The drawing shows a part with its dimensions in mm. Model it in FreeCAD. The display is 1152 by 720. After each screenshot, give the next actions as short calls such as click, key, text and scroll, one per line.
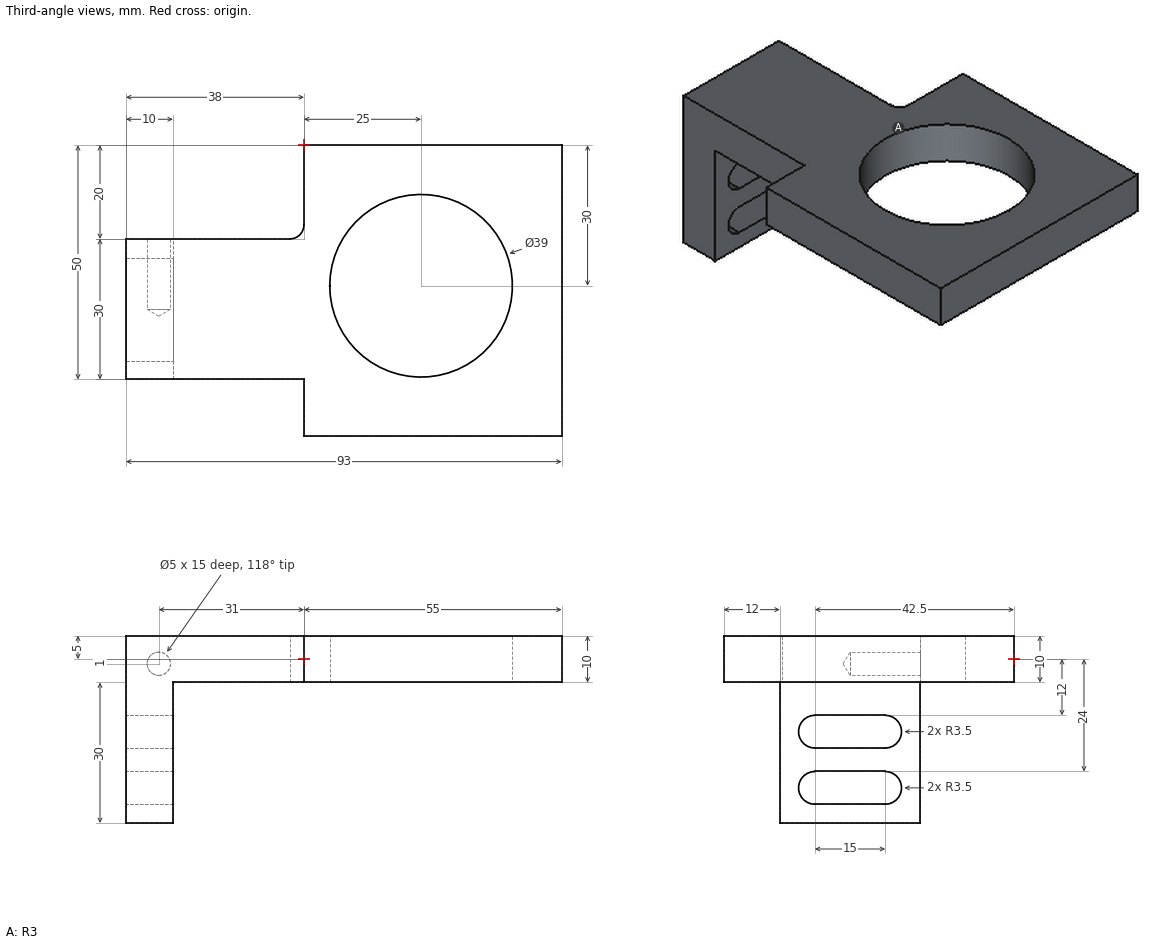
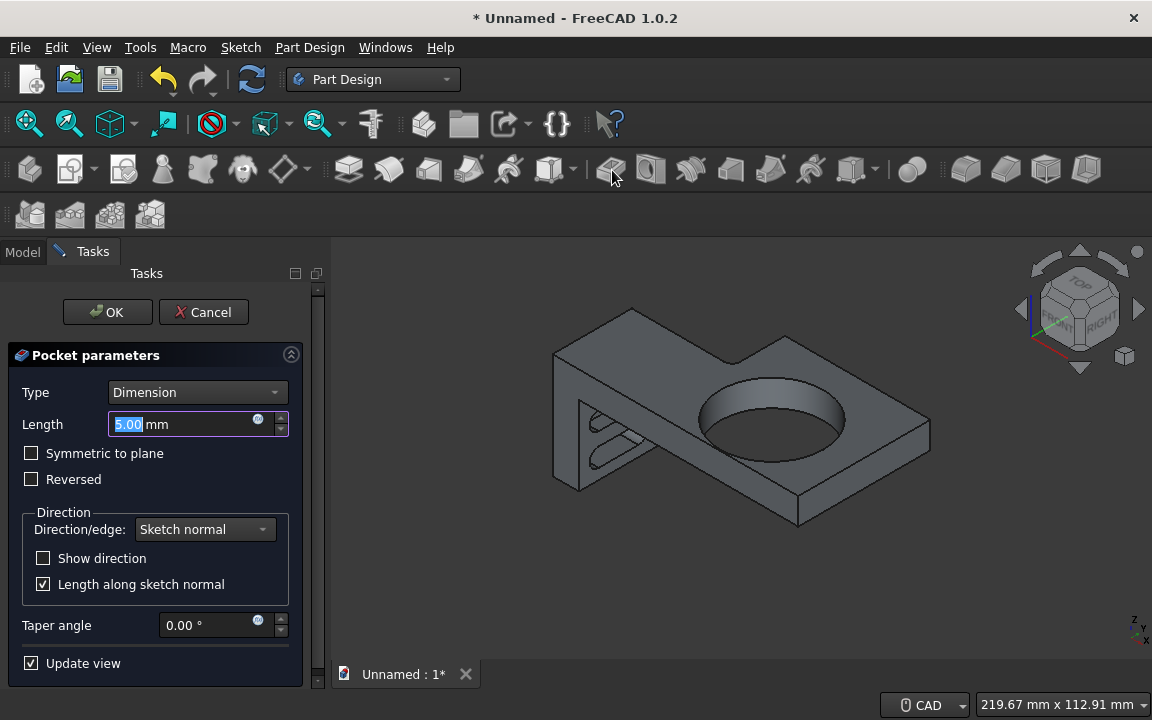
click(198, 392)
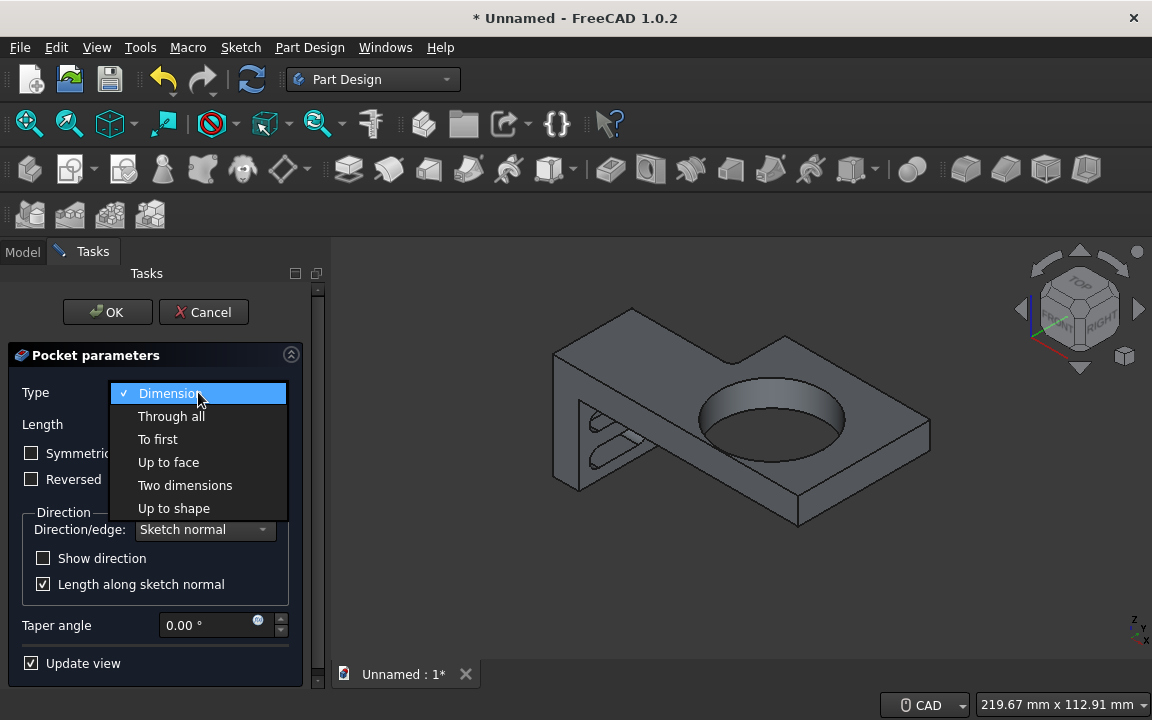
click(198, 440)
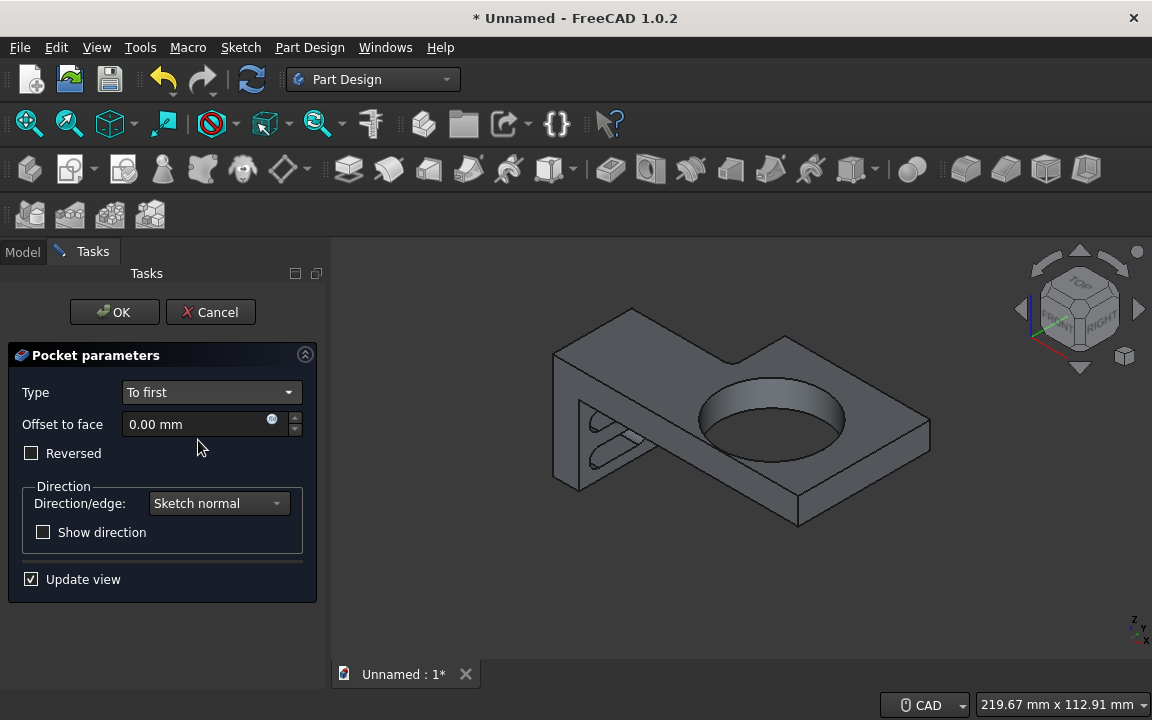
click(115, 312)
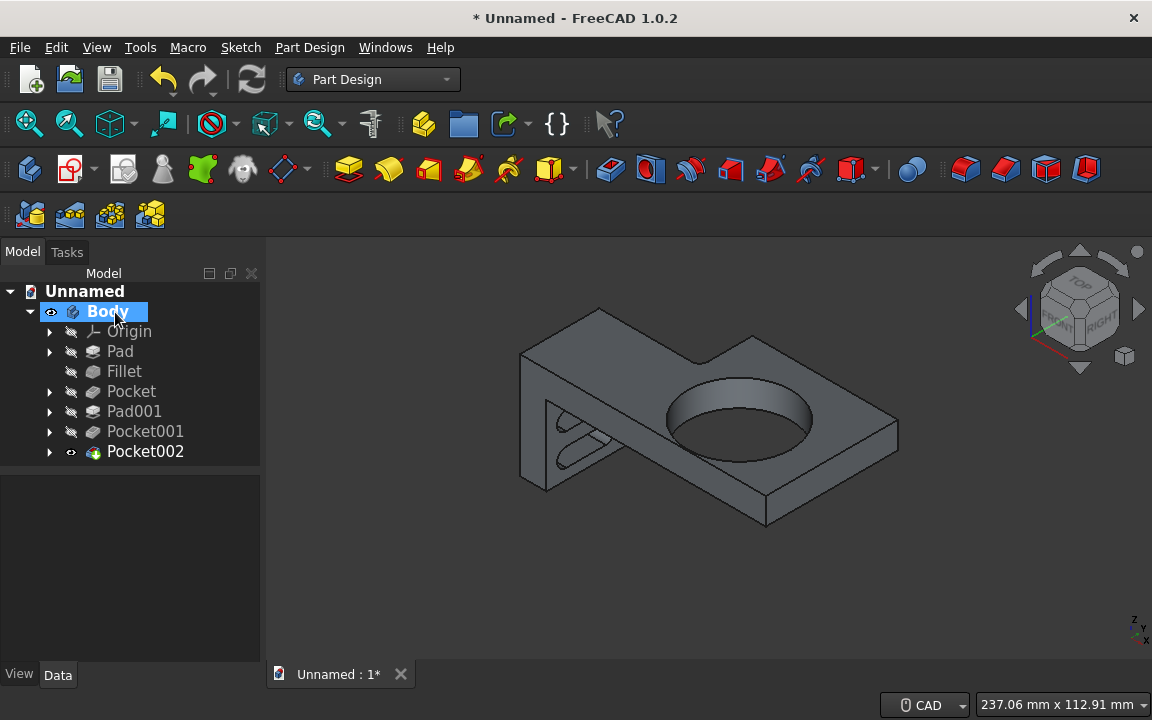
key(4)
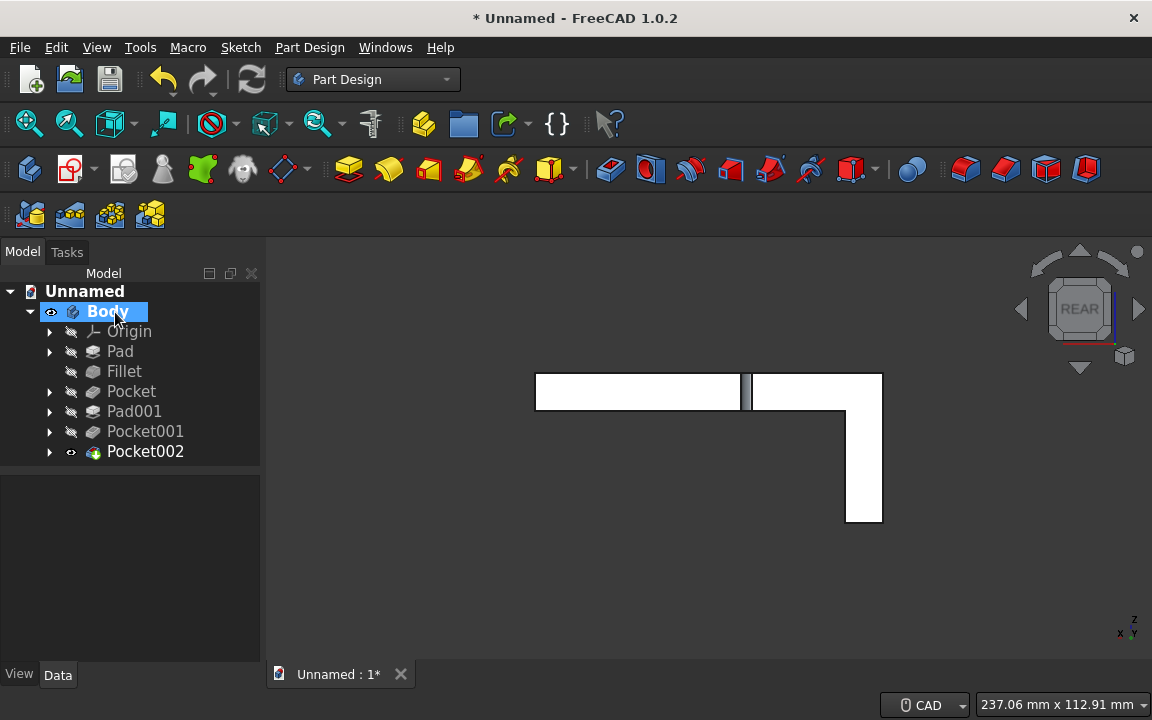
key(v)
key(f)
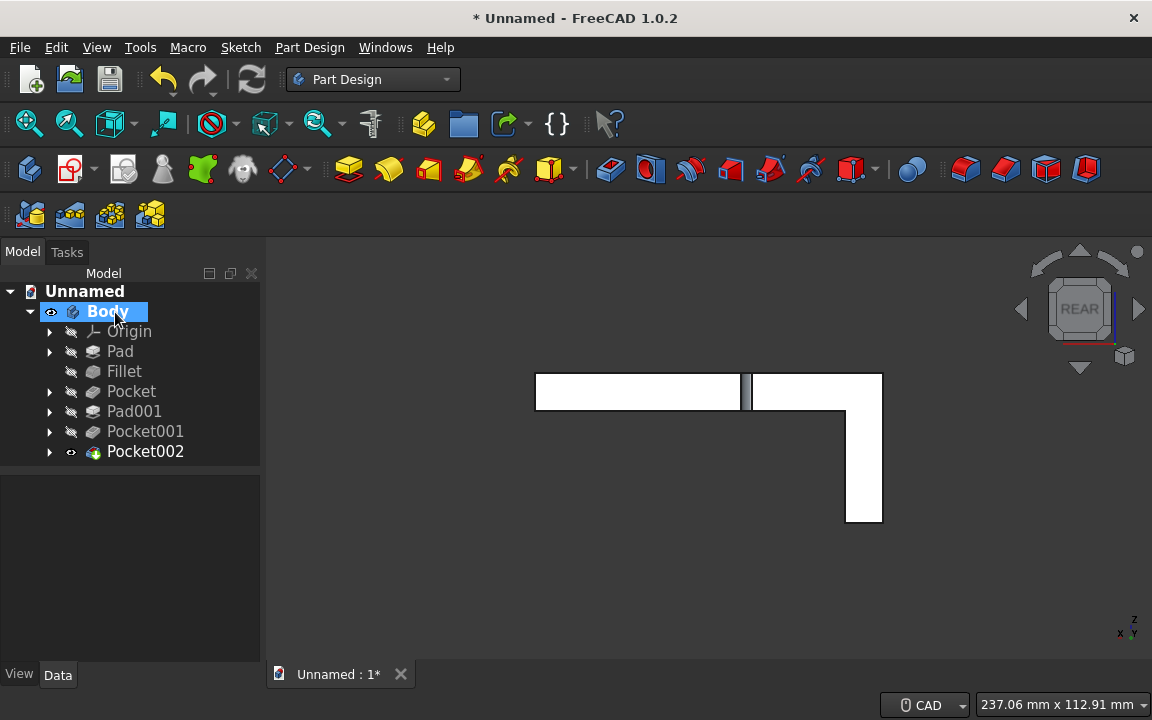
click(855, 404)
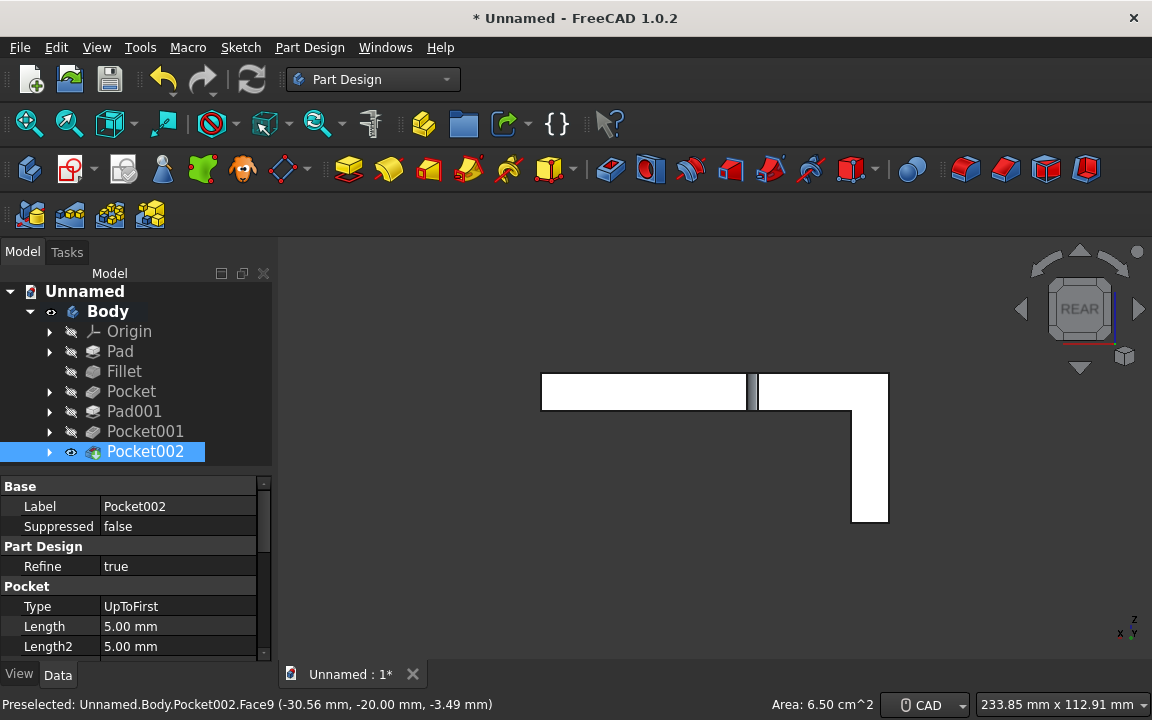
click(70, 170)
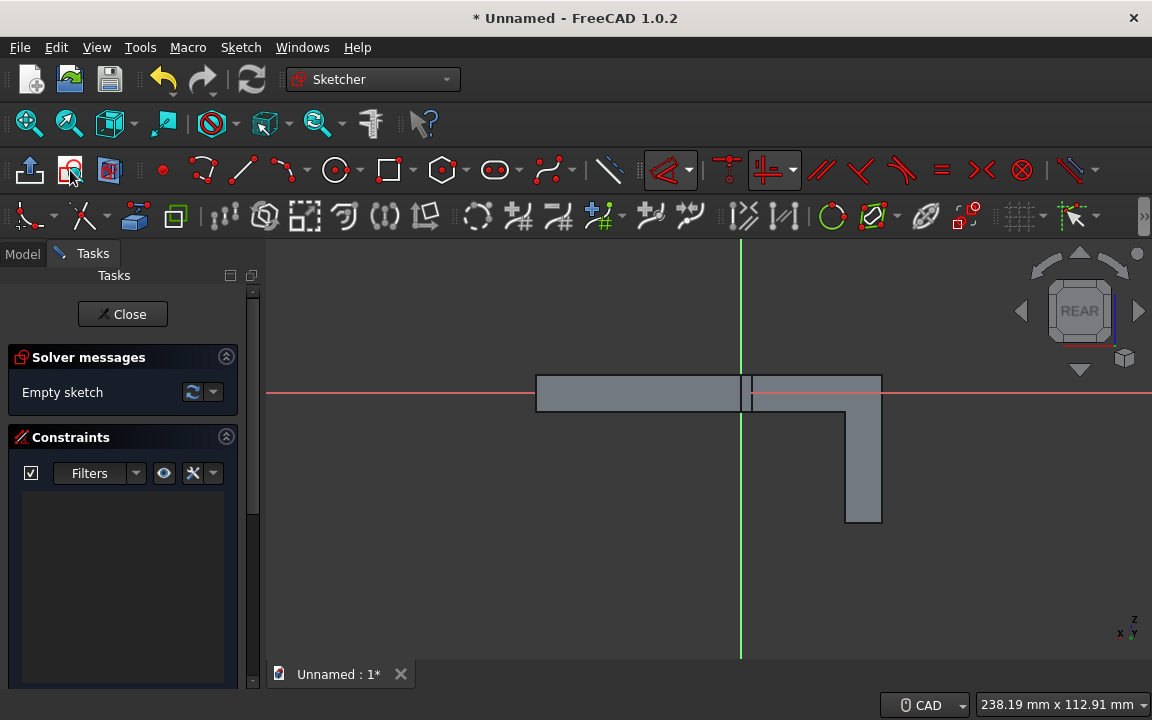
scroll(873, 393, up, 13)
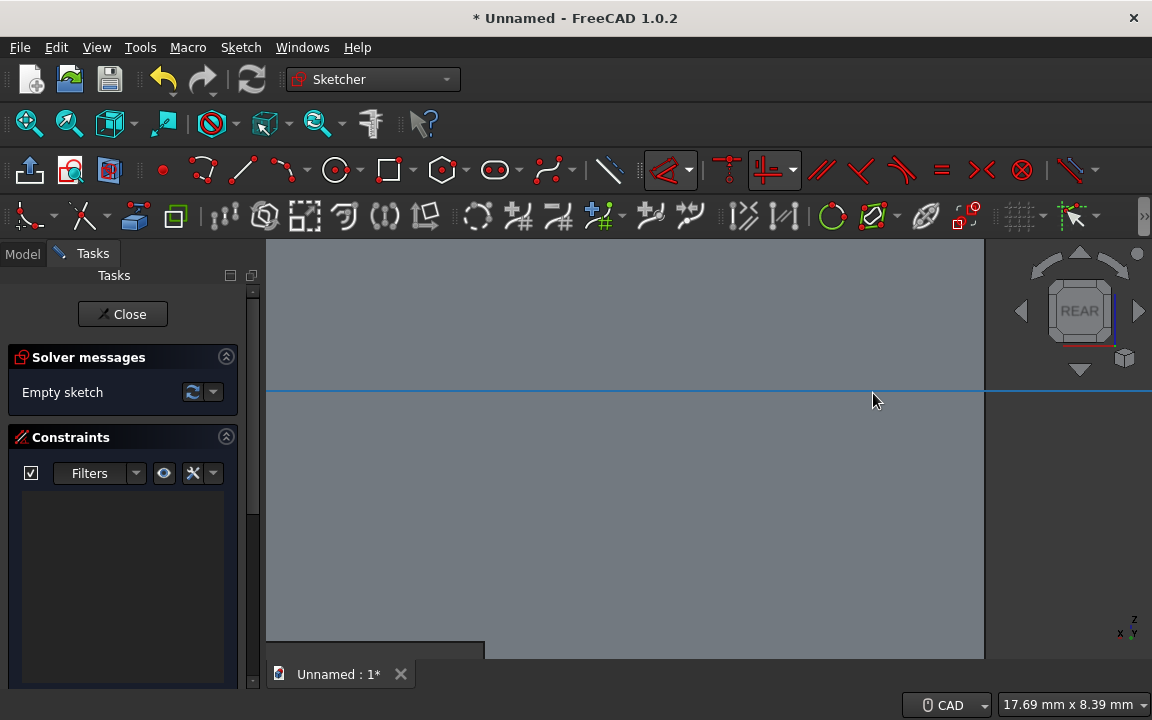
click(336, 170)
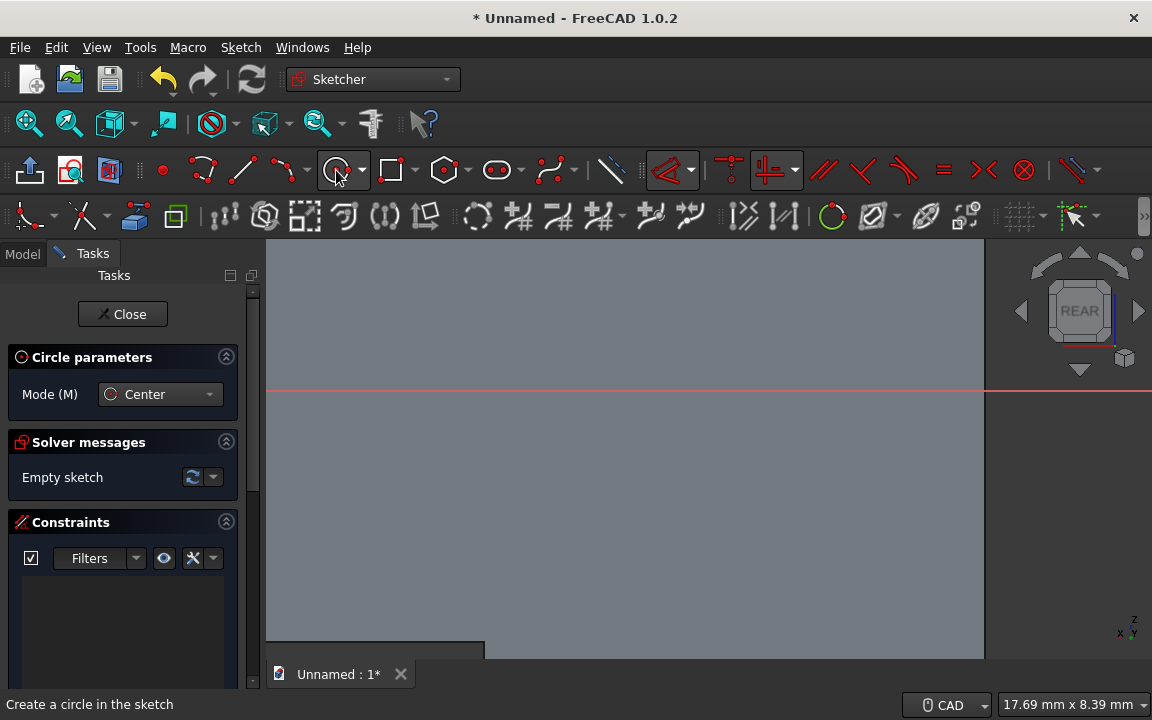
click(635, 441)
move(723, 353)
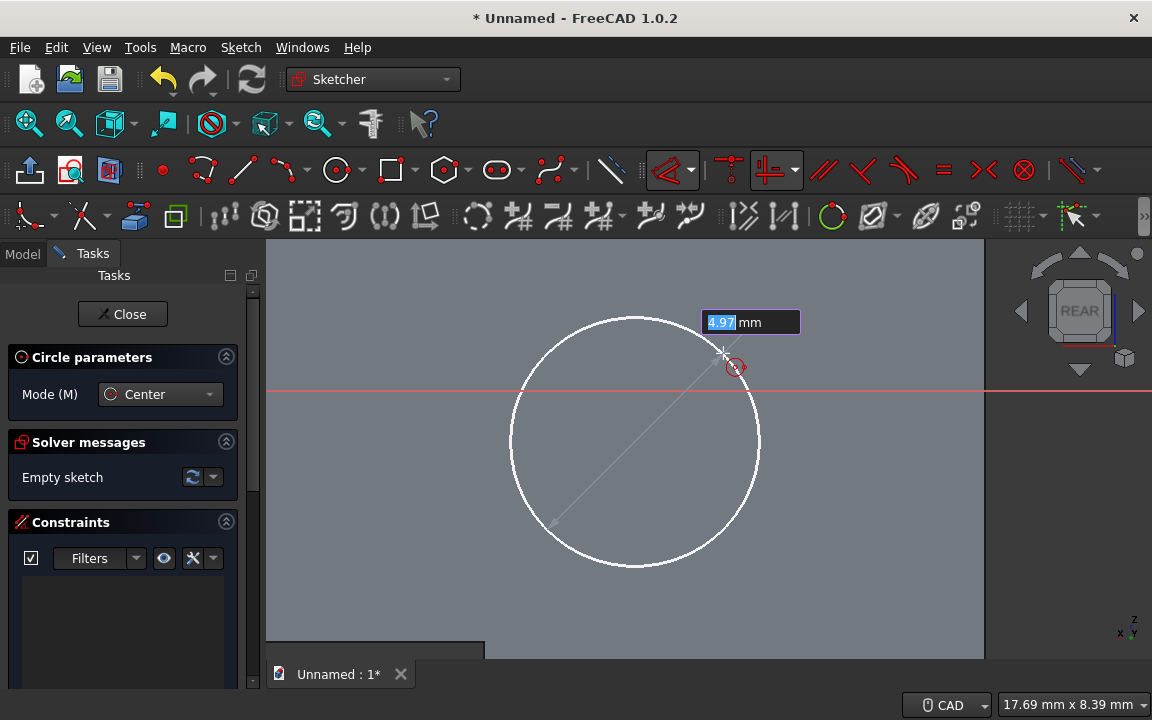
text(5)
key(Return)
key(Escape)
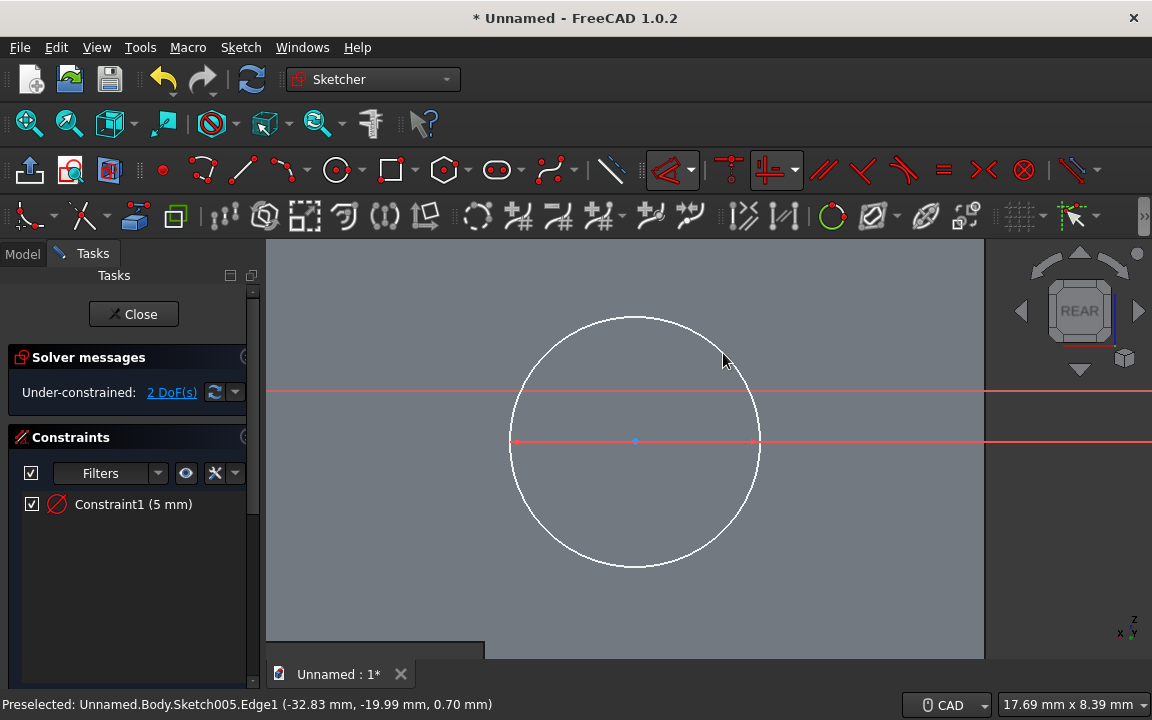
click(635, 442)